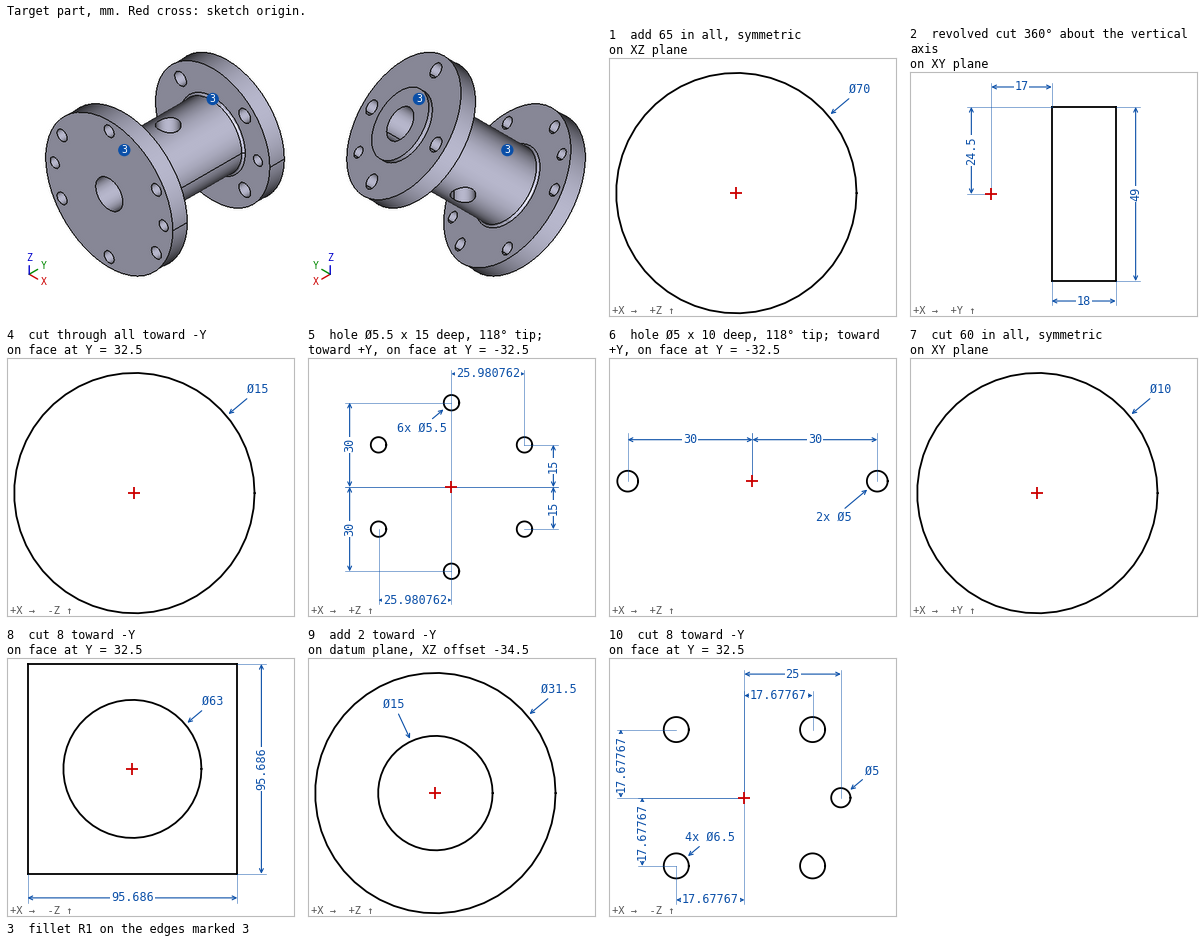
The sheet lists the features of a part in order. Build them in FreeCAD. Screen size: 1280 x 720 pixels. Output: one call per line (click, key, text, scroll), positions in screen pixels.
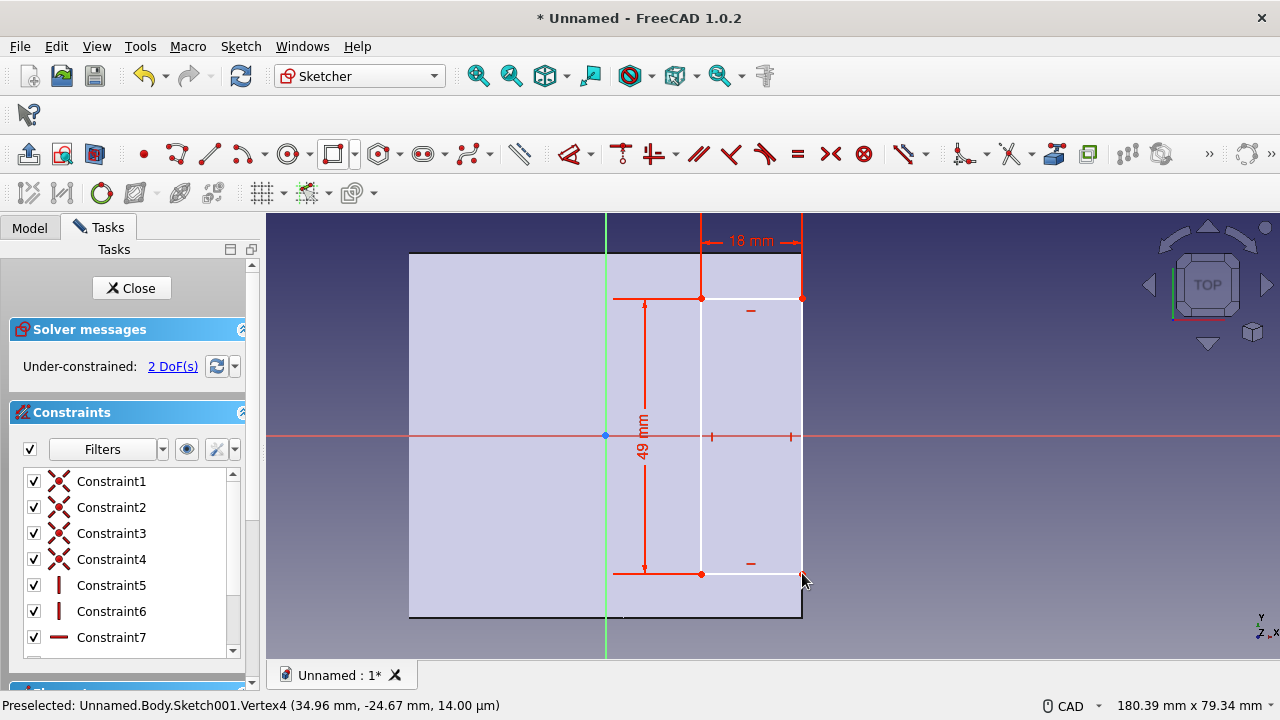
click(568, 154)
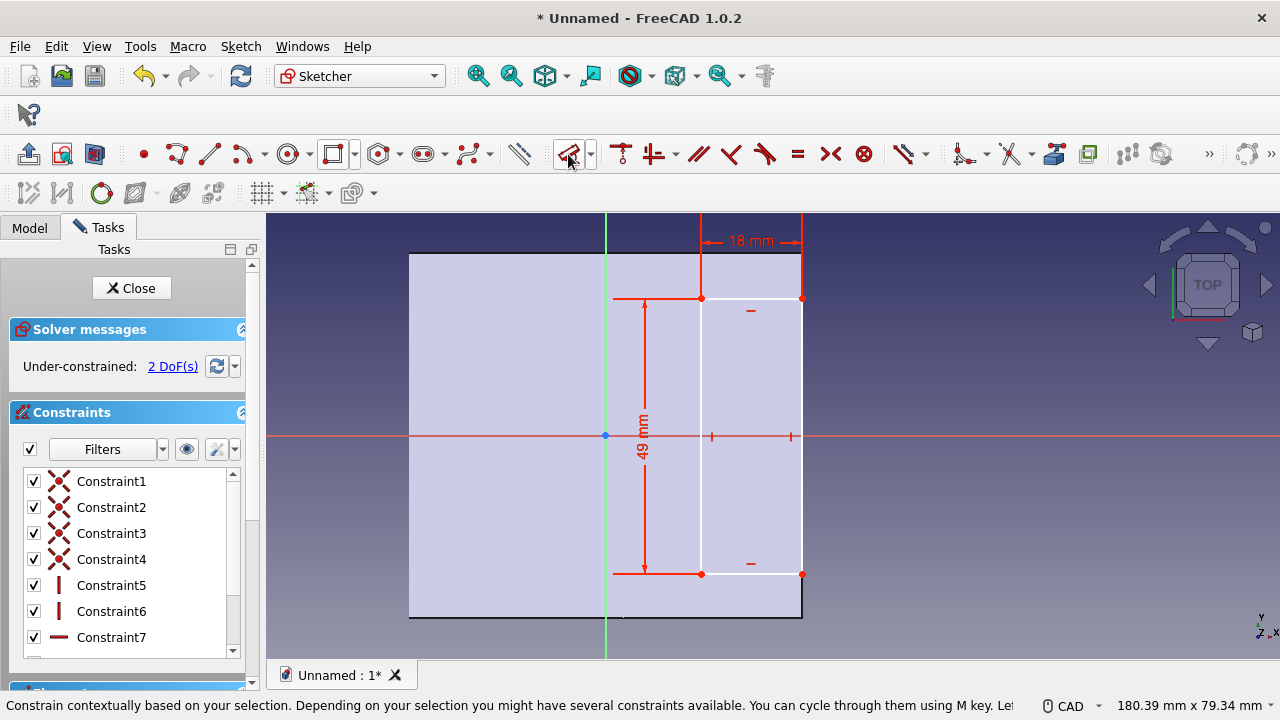
click(701, 299)
click(653, 265)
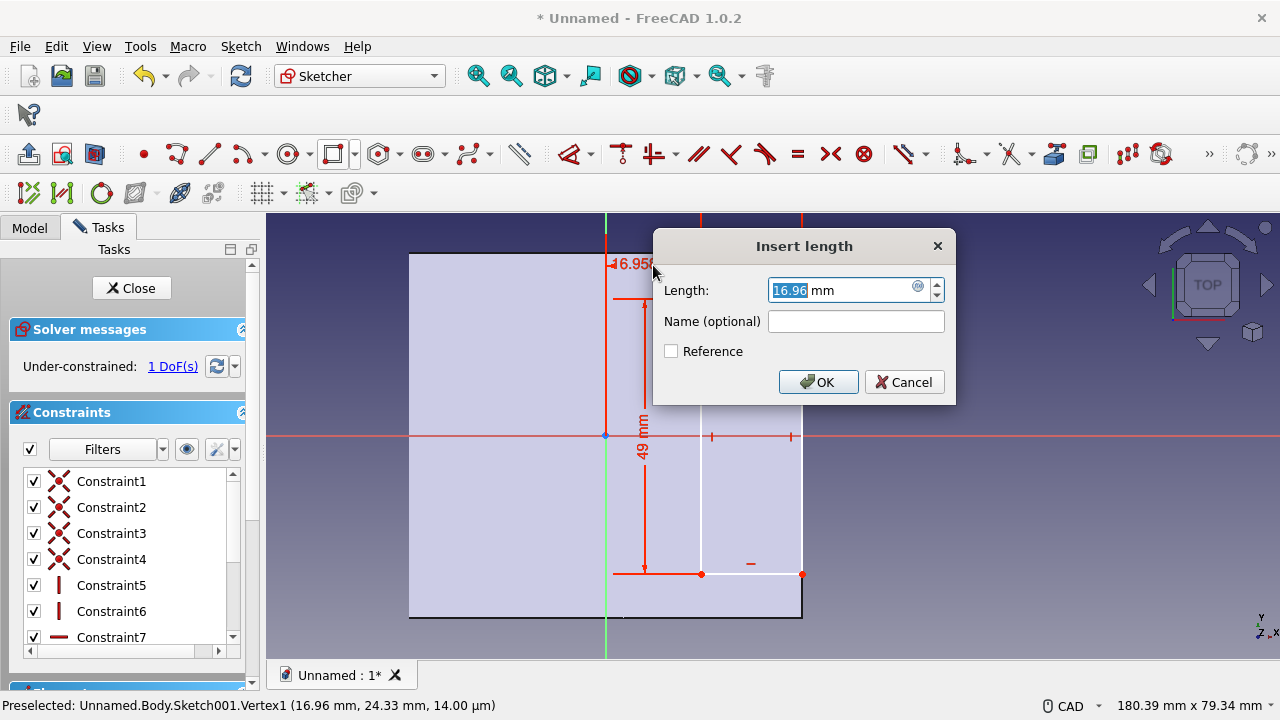
text(17)
key(Return)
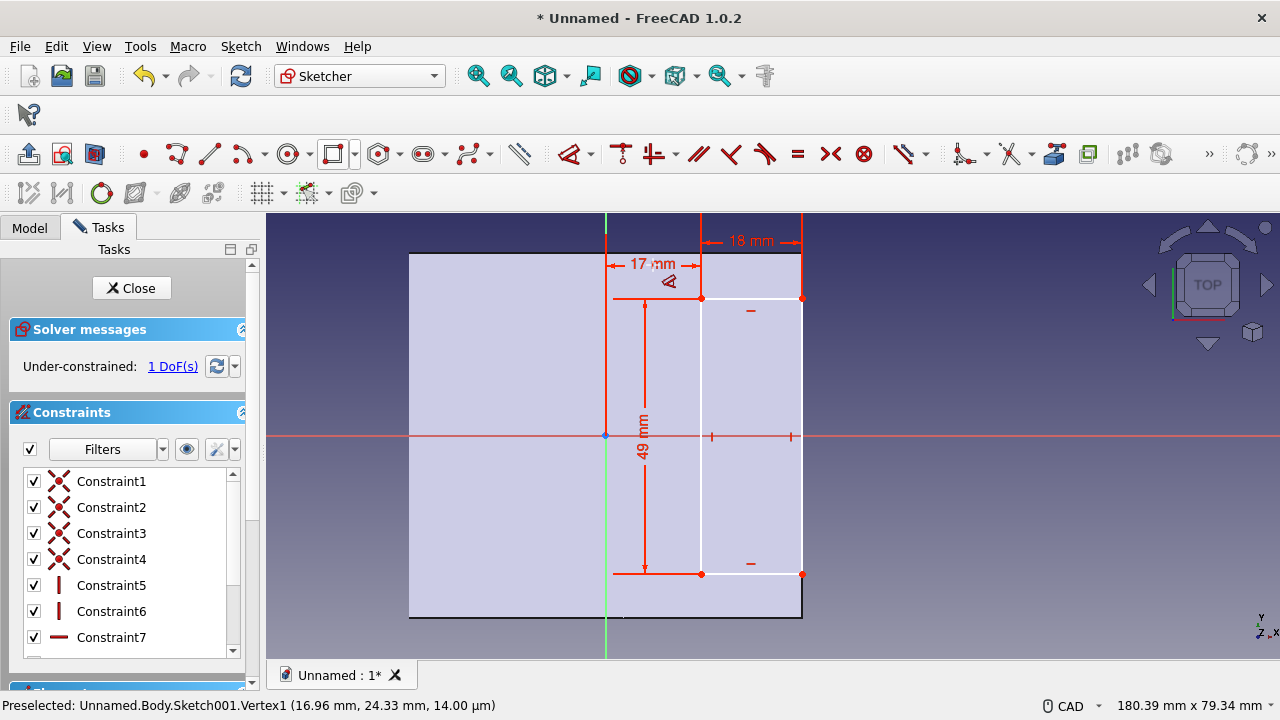
click(701, 299)
click(572, 367)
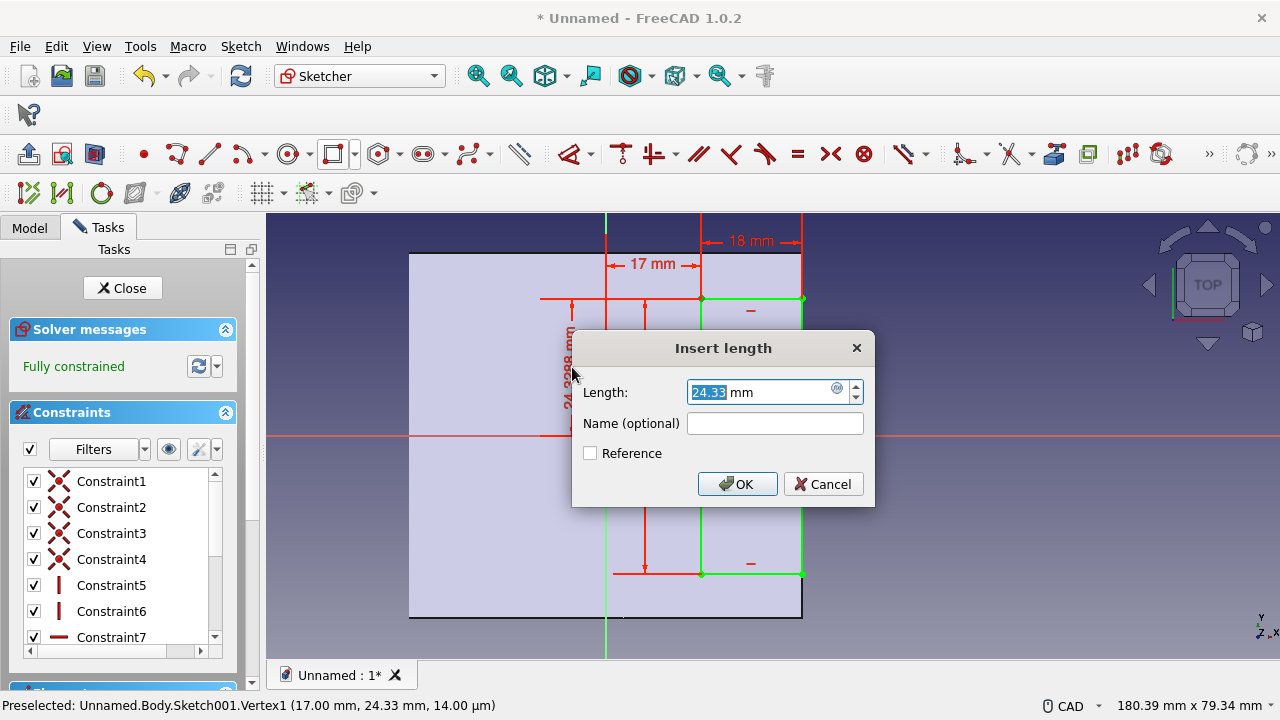
text(24.5)
key(Return)
key(Escape)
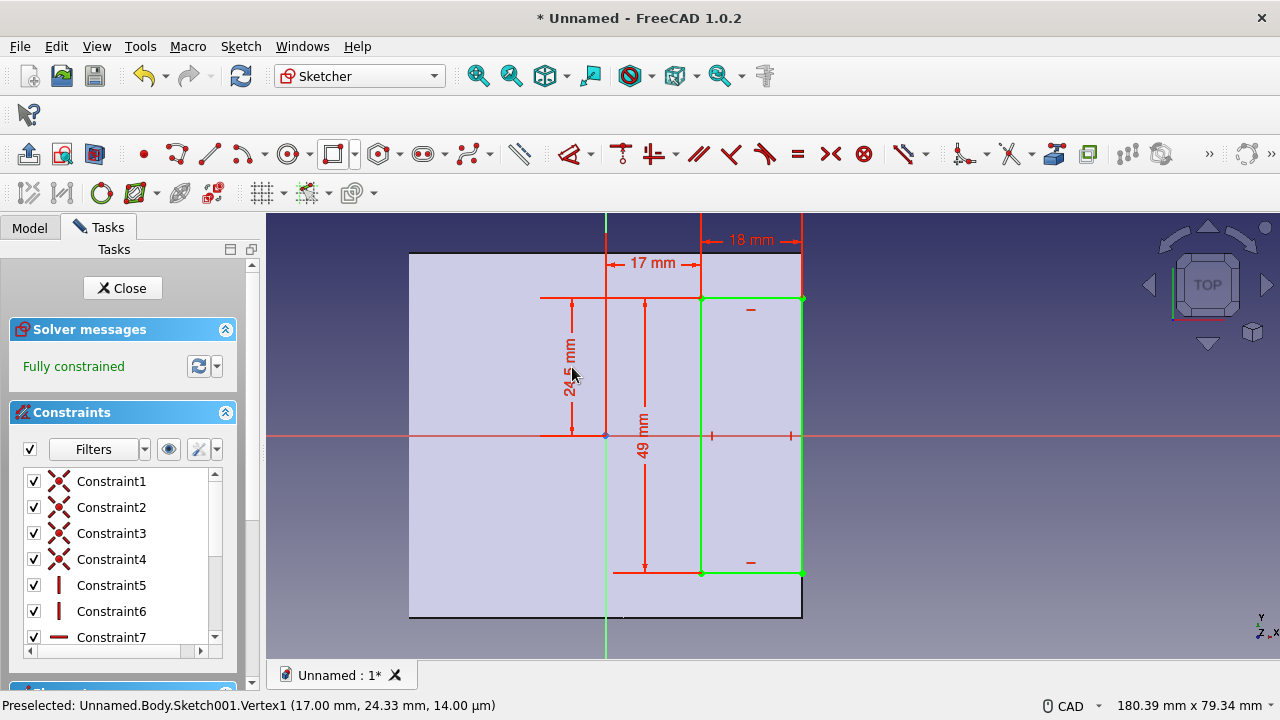
click(123, 288)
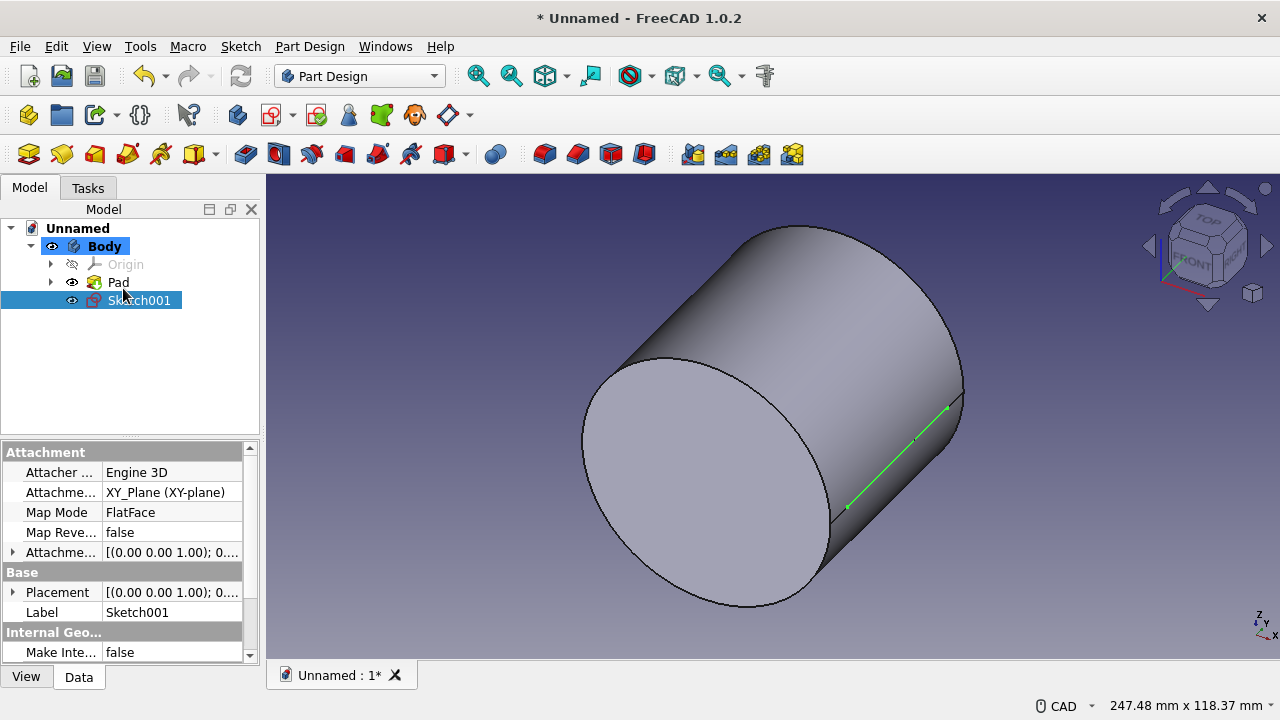
click(312, 154)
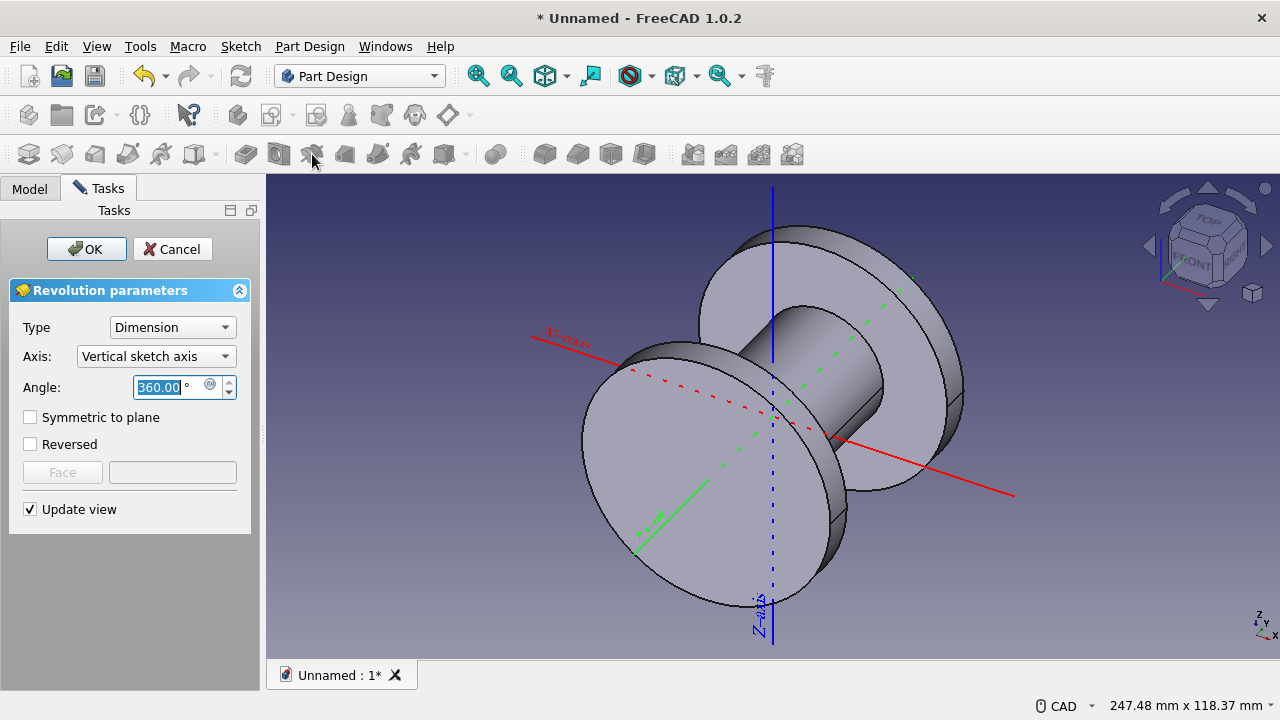
click(87, 249)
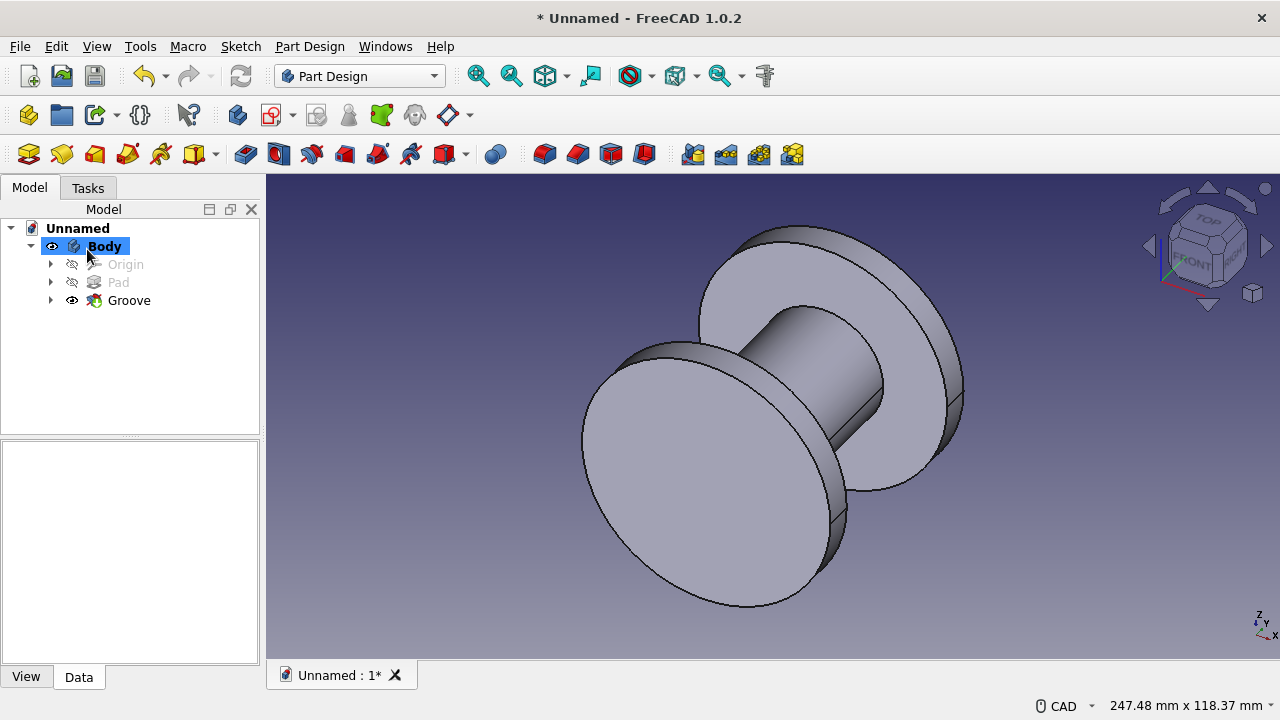
key(0)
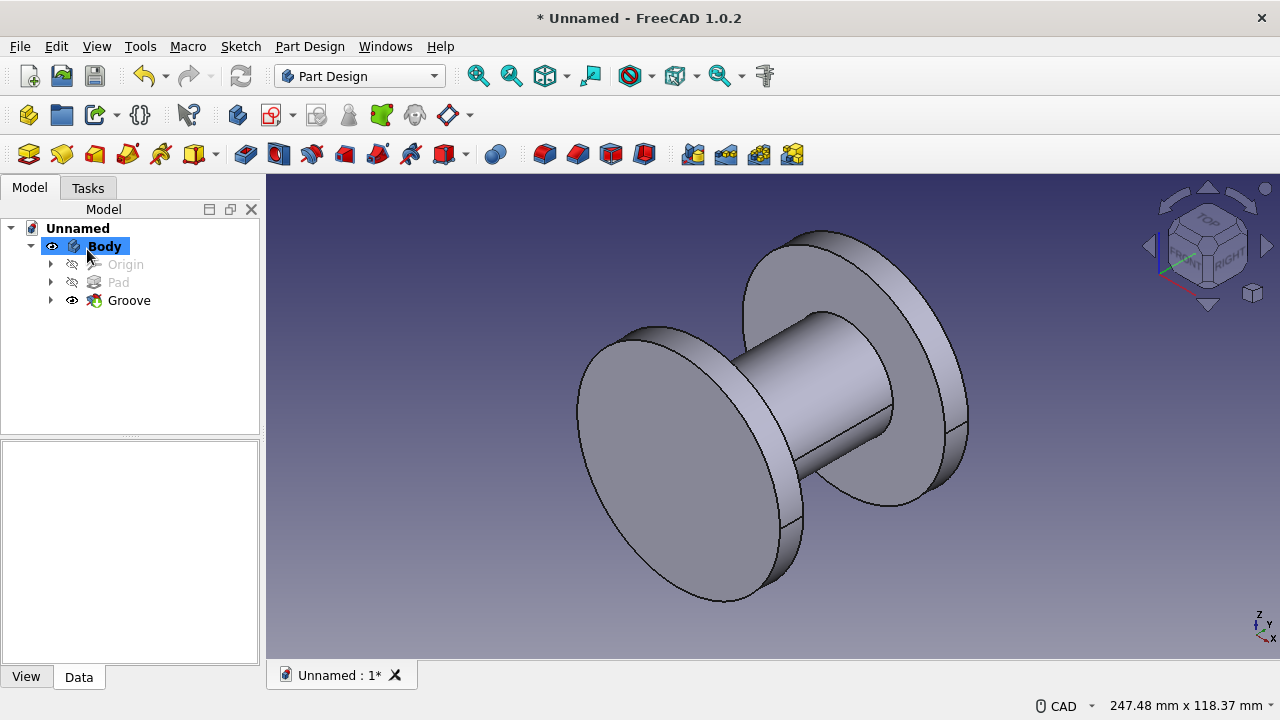
key(2)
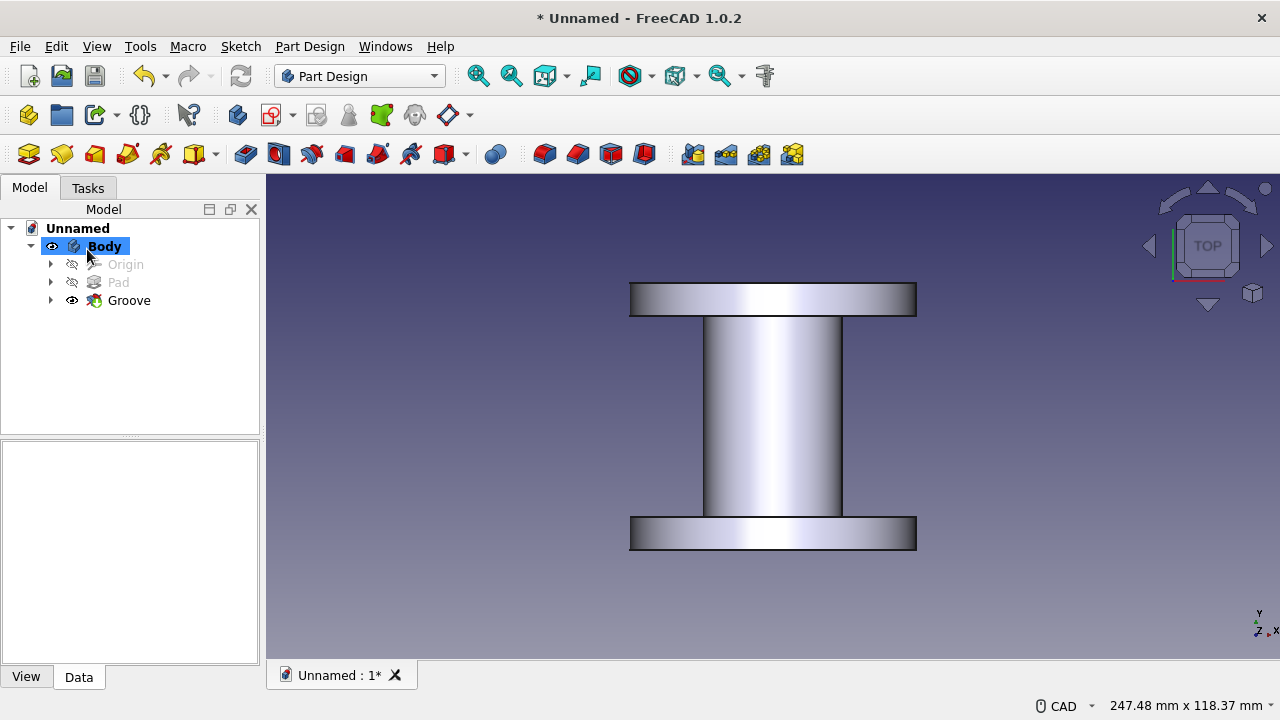
key(1)